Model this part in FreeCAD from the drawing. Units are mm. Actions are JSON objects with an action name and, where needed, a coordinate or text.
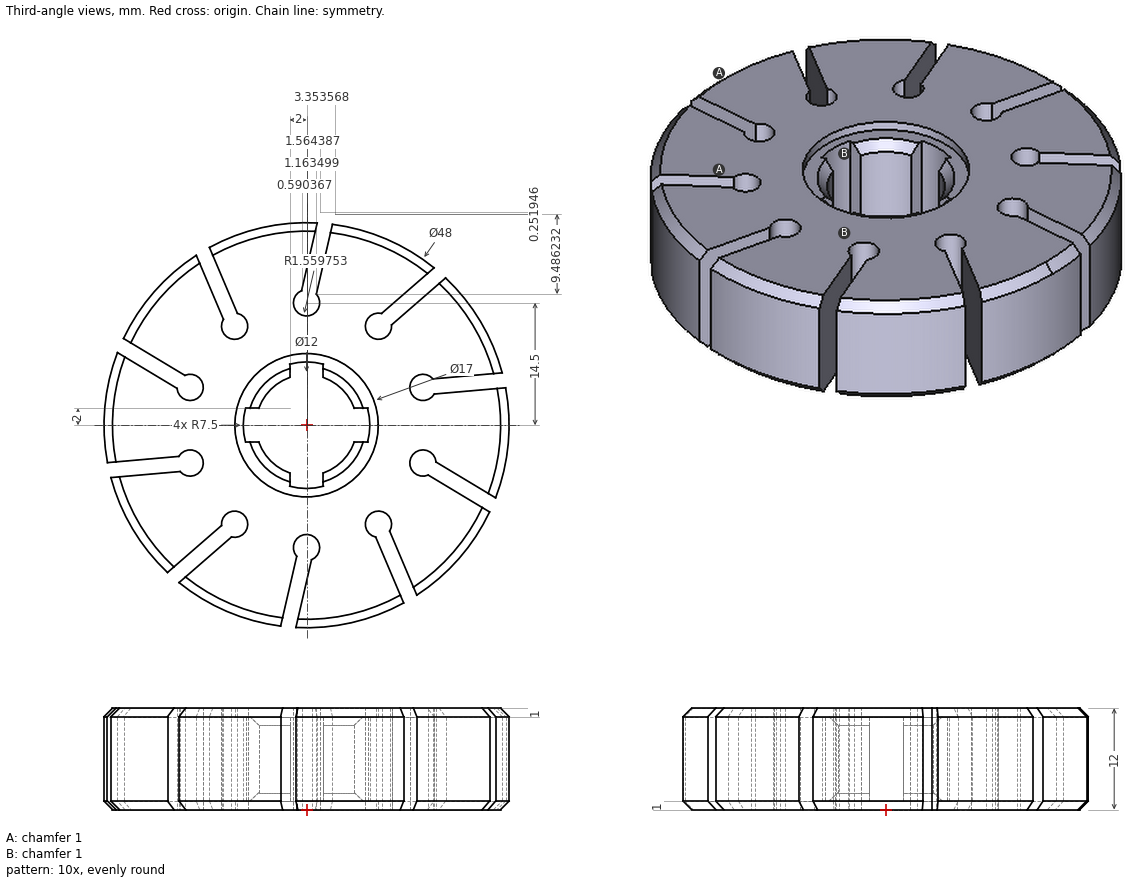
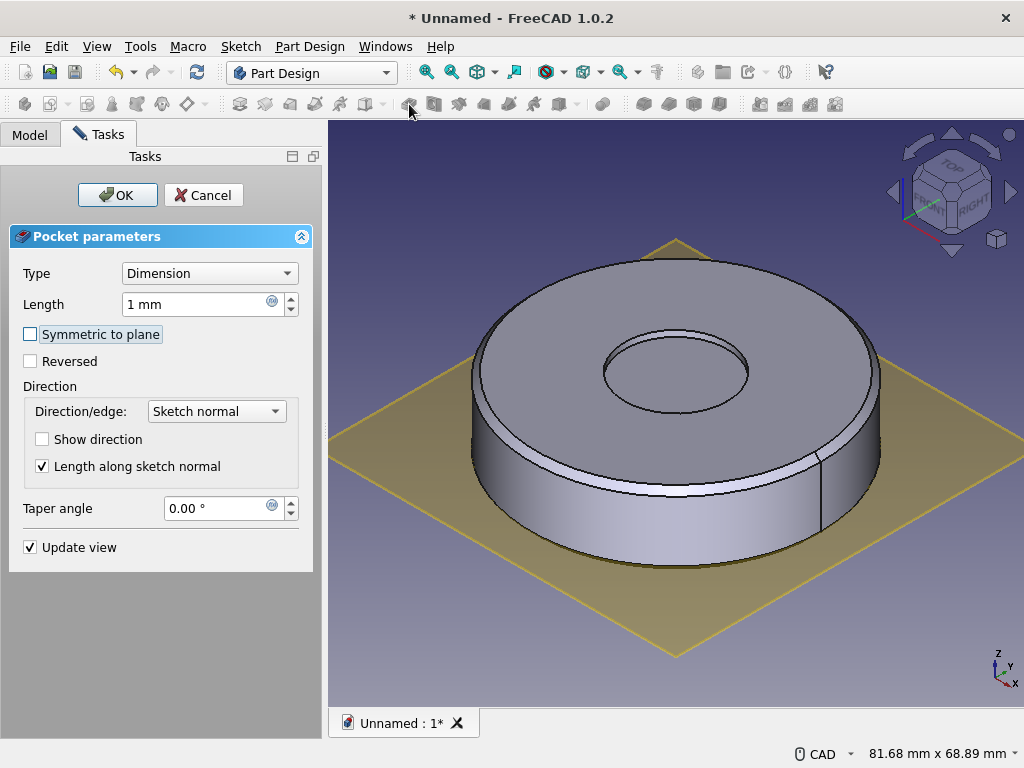
{"action": "left_click", "coordinate": [118, 195]}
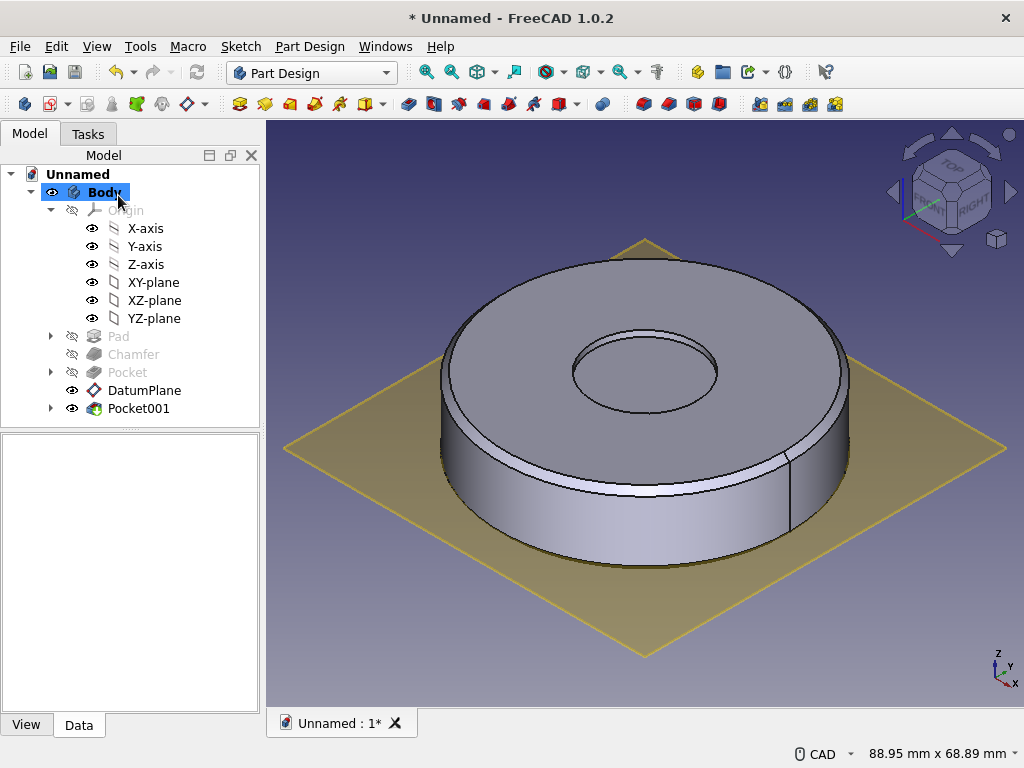
{"action": "left_click", "coordinate": [117, 390]}
{"action": "key", "text": "space"}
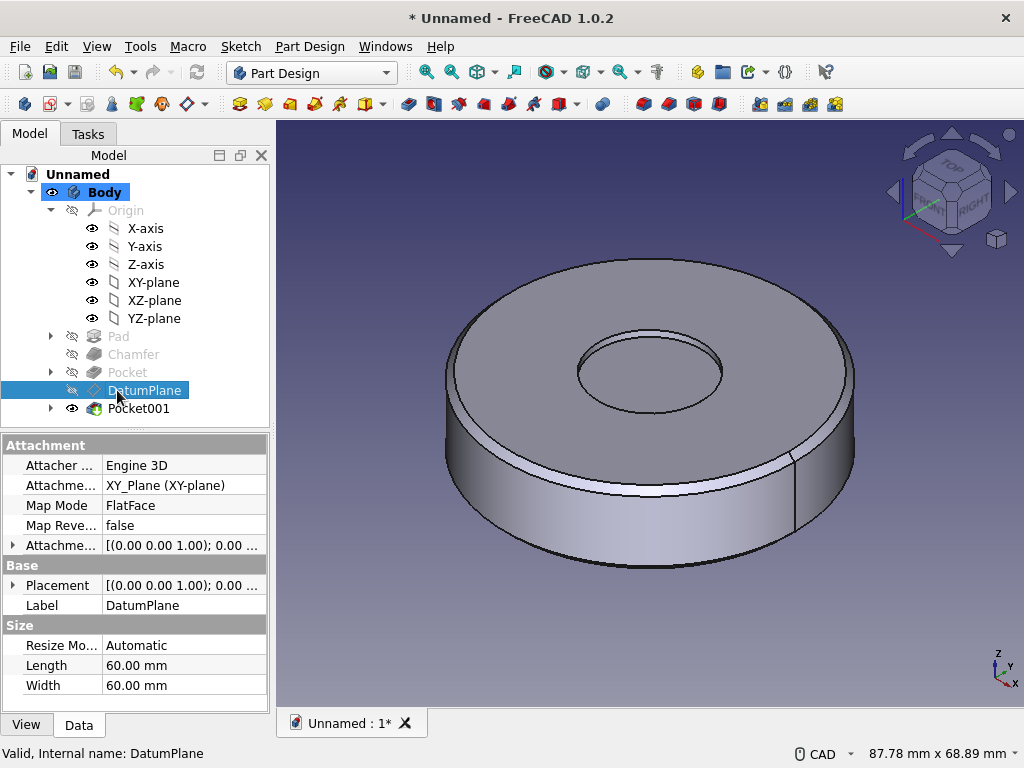
{"action": "left_click", "coordinate": [650, 378]}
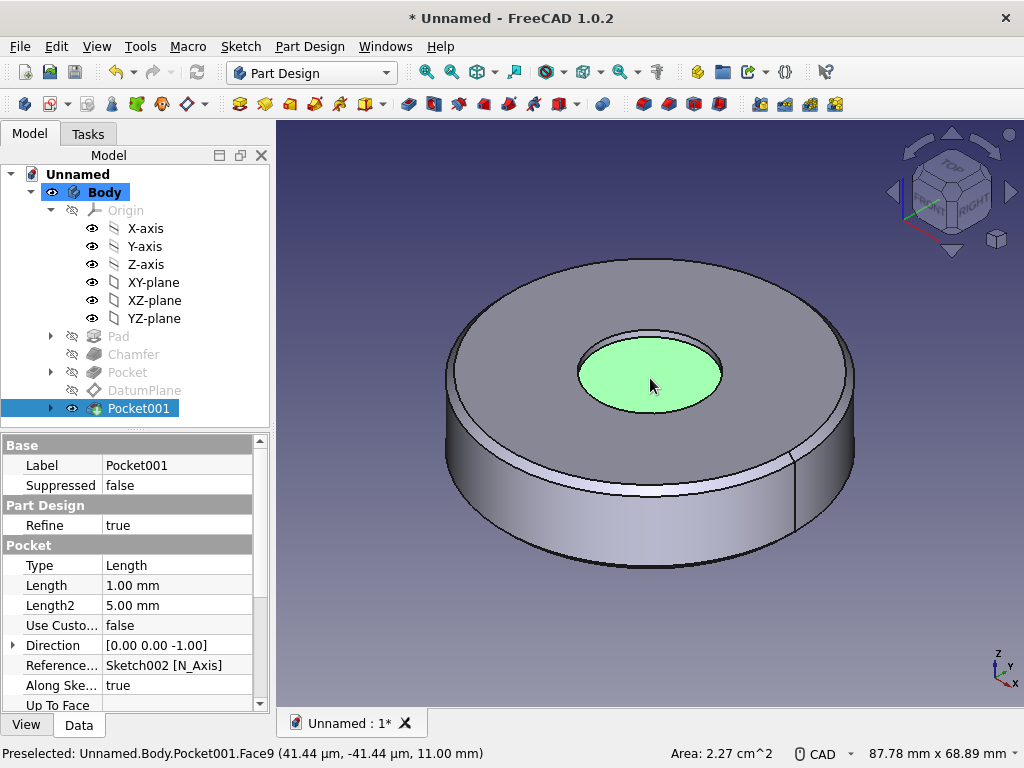
{"action": "left_click", "coordinate": [50, 104]}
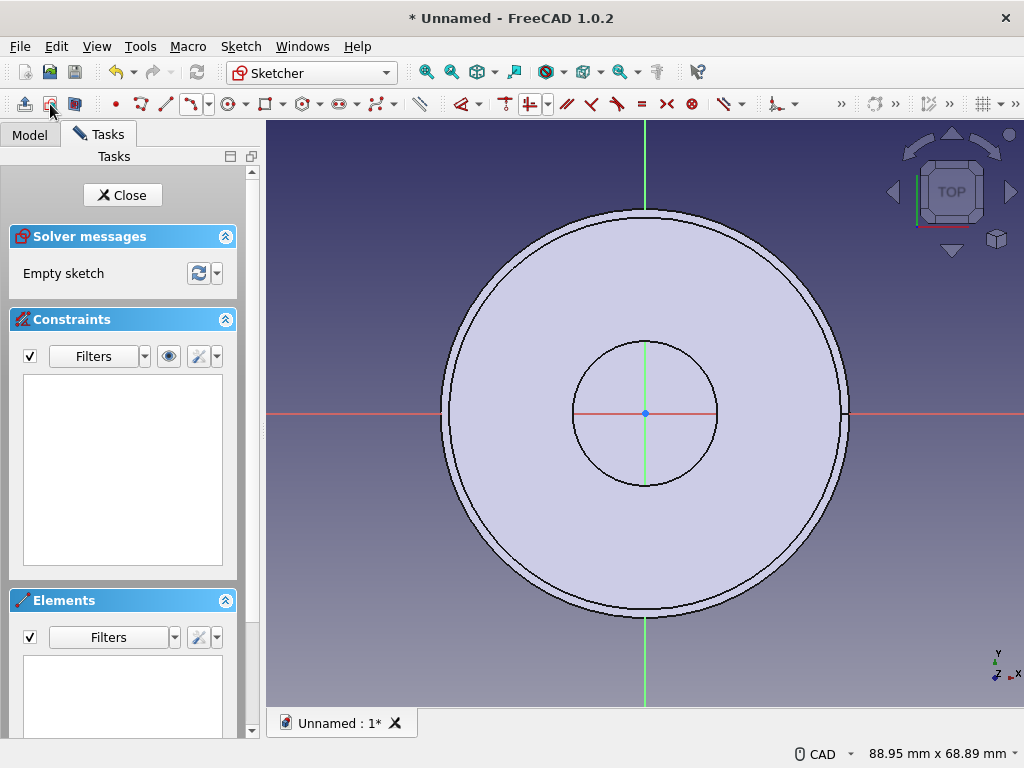
{"action": "left_click", "coordinate": [75, 104]}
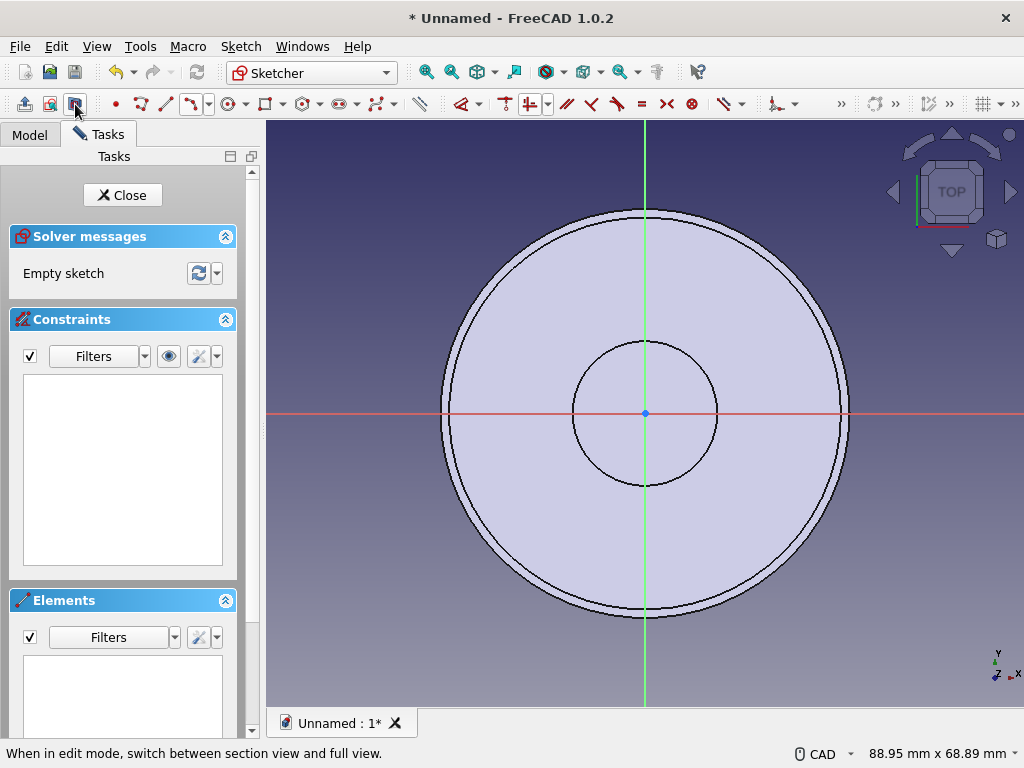
{"action": "scroll", "coordinate": [675, 413], "scroll_direction": "up", "scroll_amount": 6}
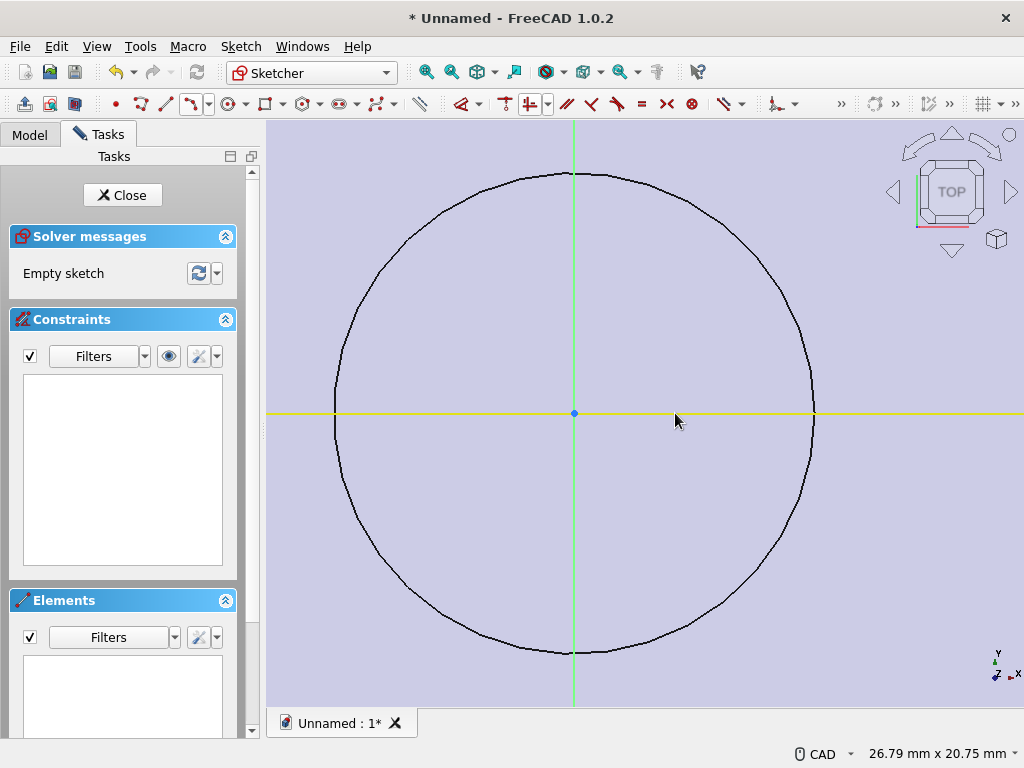
{"action": "left_click", "coordinate": [228, 104]}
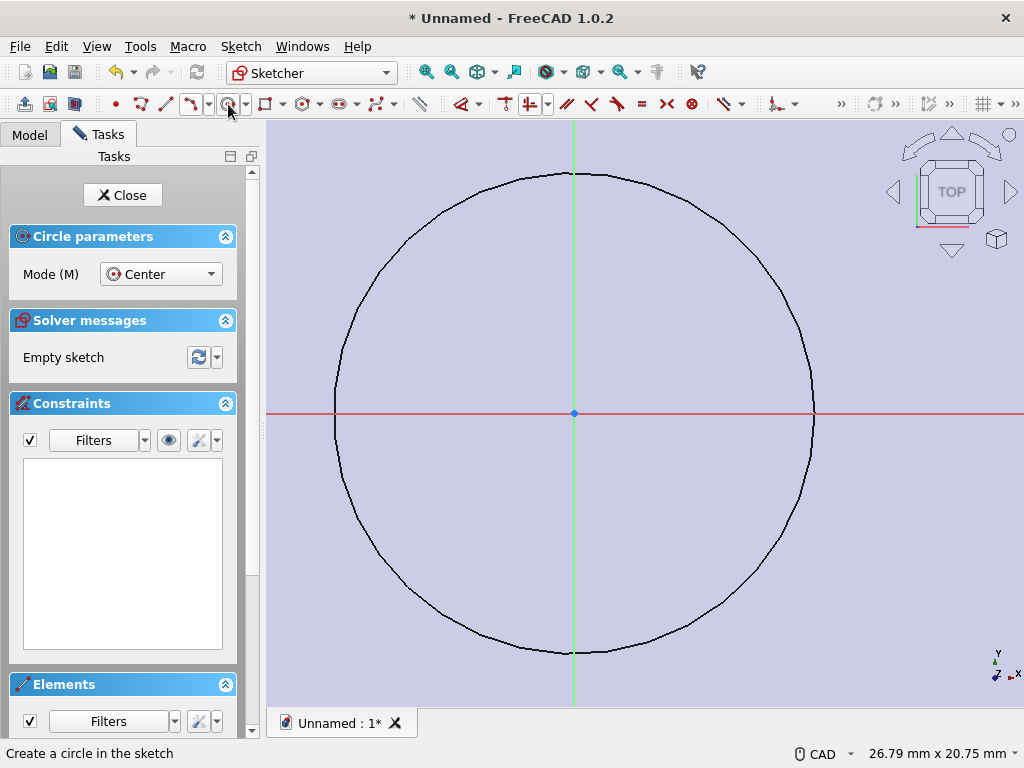
{"action": "left_click", "coordinate": [574, 413]}
{"action": "mouse_move", "coordinate": [694, 293]}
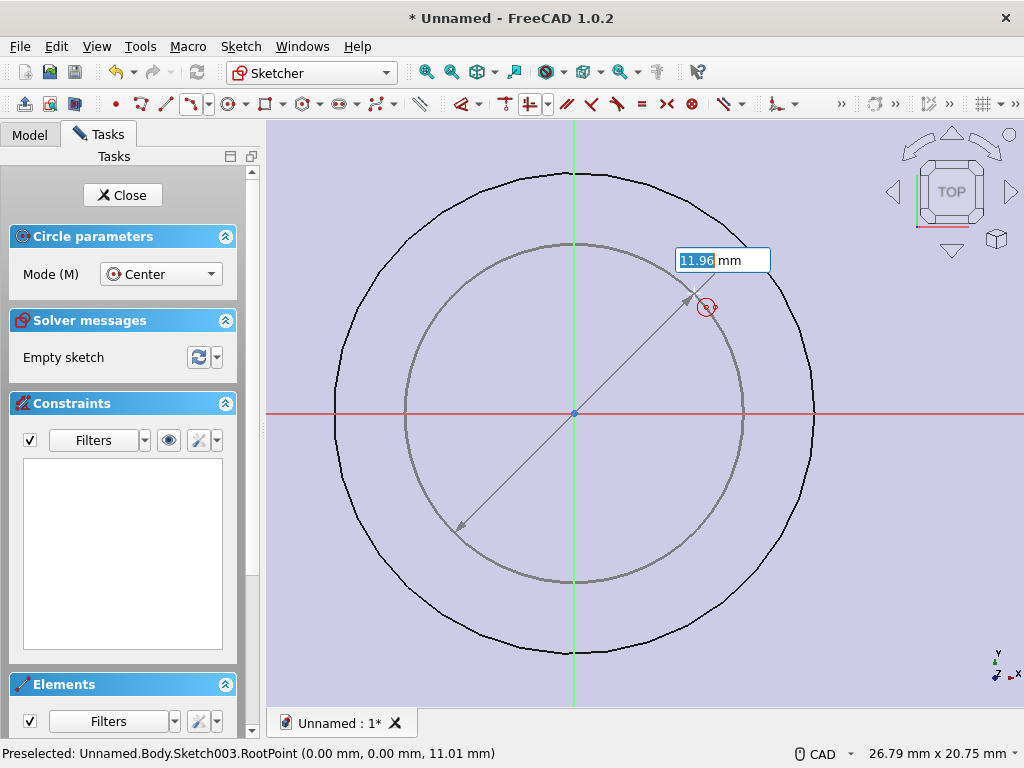
{"action": "type", "text": "12"}
{"action": "key", "text": "Return"}
{"action": "key", "text": "Escape"}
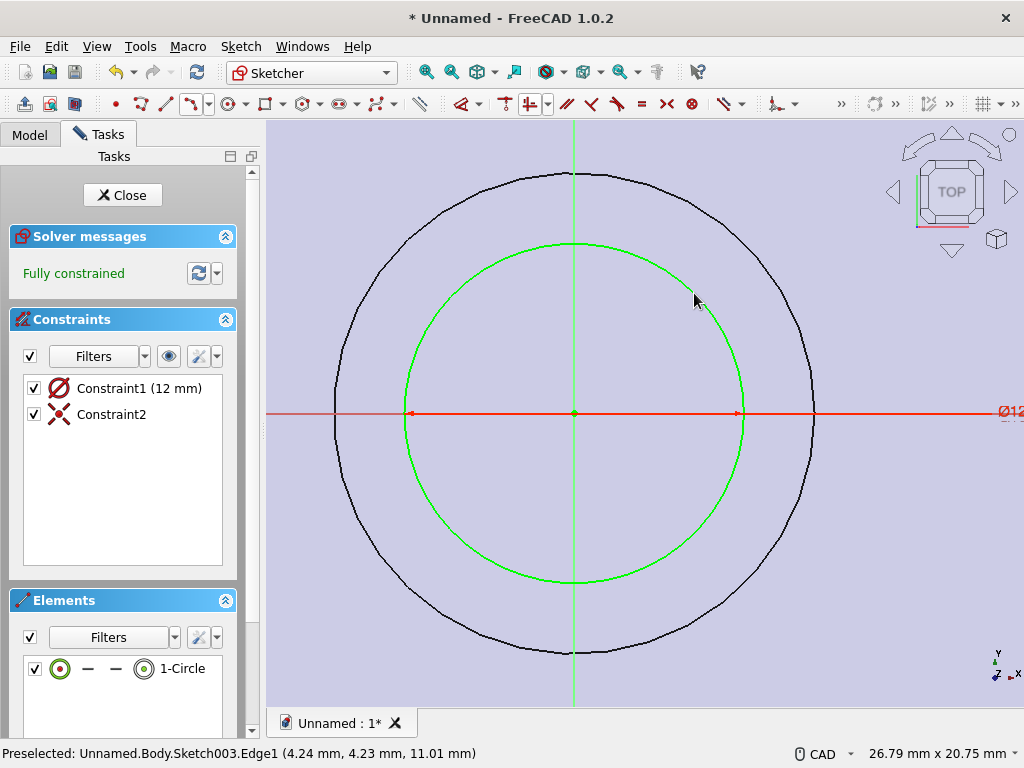
{"action": "left_click", "coordinate": [123, 195]}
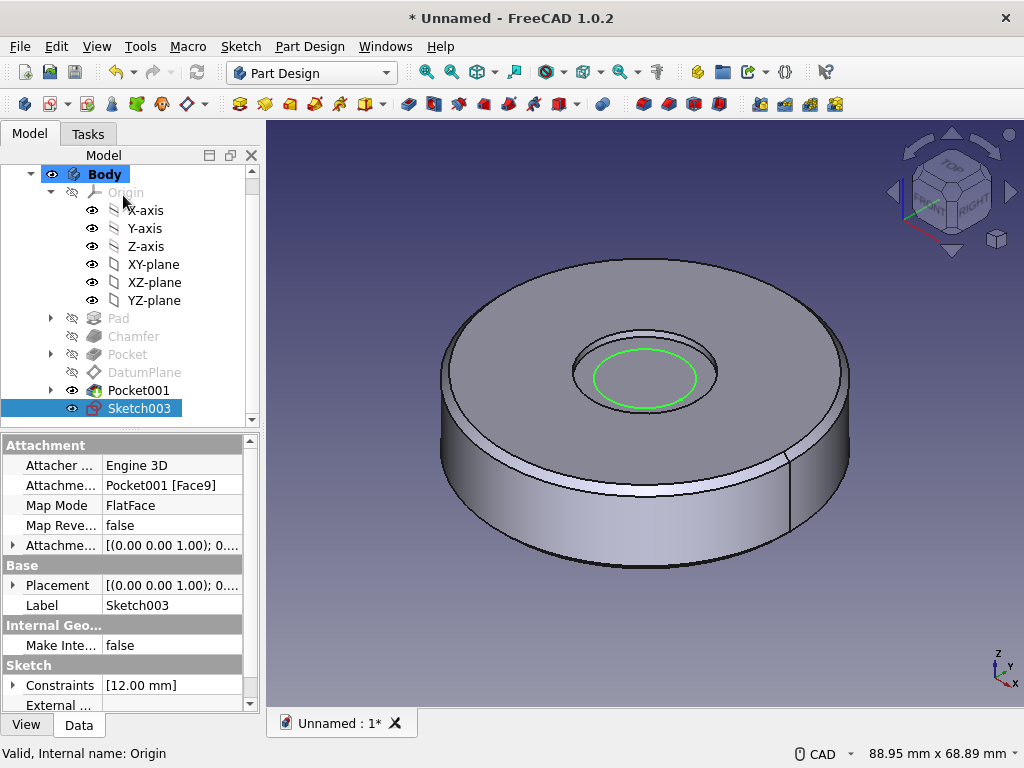
{"action": "left_click", "coordinate": [409, 104]}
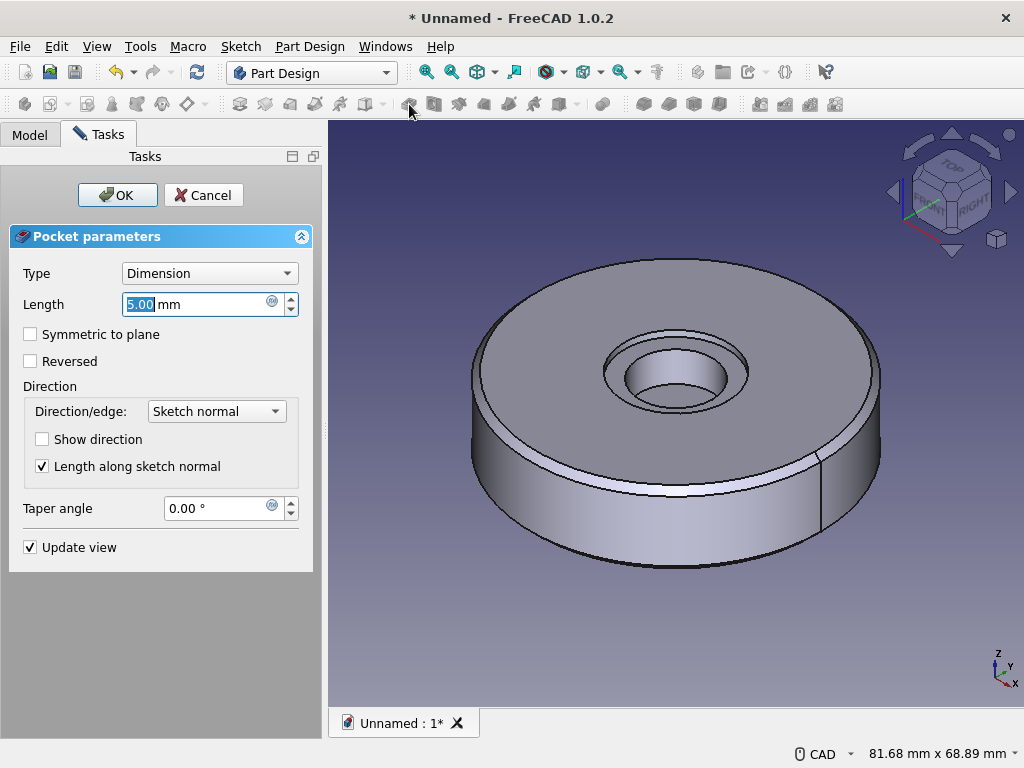
{"action": "left_click", "coordinate": [210, 274]}